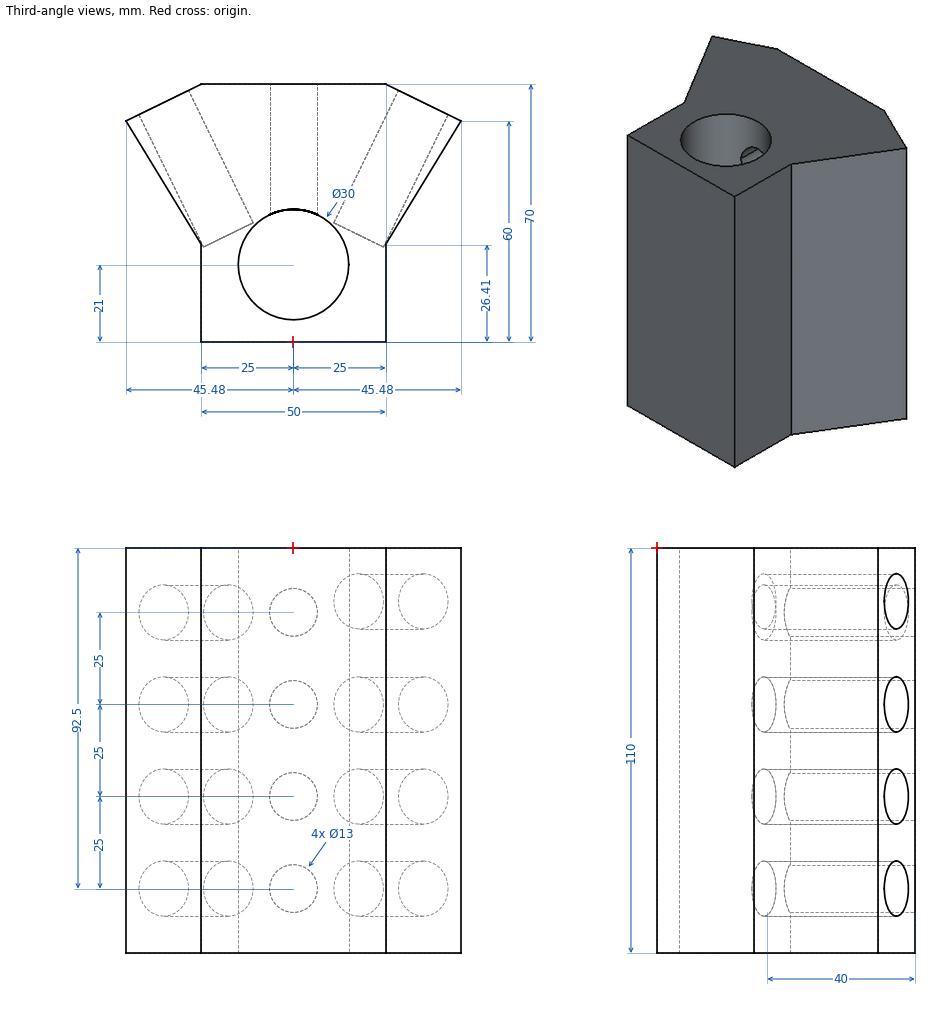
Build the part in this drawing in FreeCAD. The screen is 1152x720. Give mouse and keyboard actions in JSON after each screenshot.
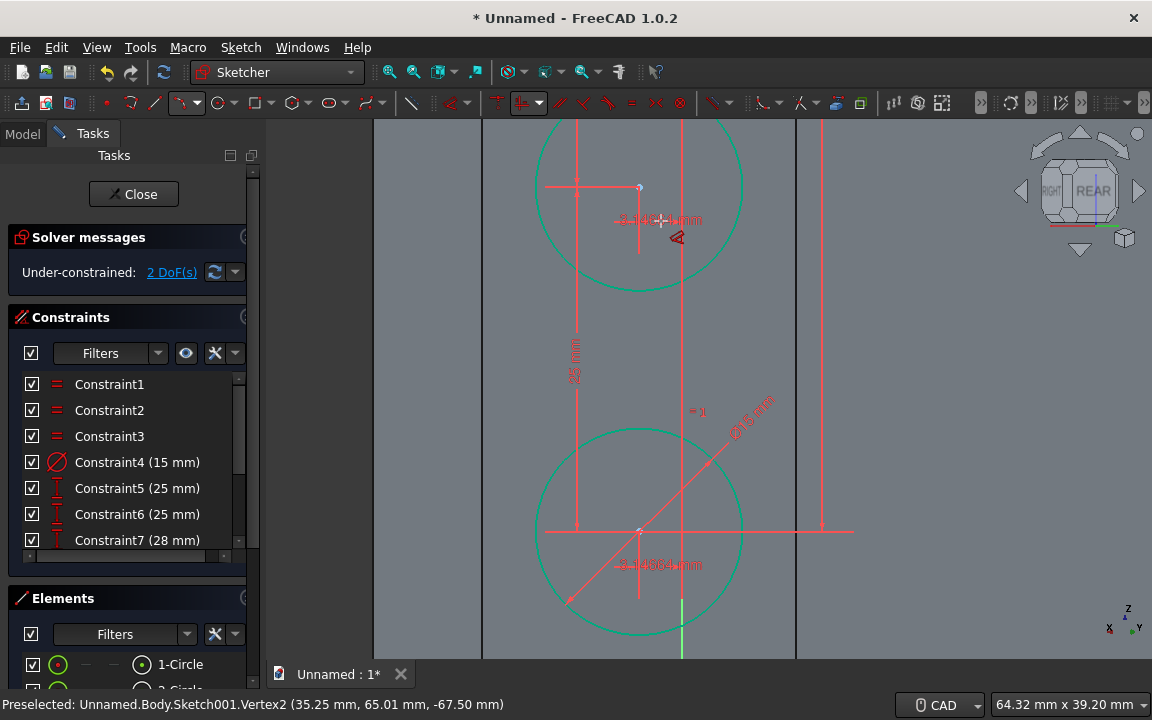
{"action": "scroll", "coordinate": [641, 534], "scroll_direction": "down", "scroll_amount": 7}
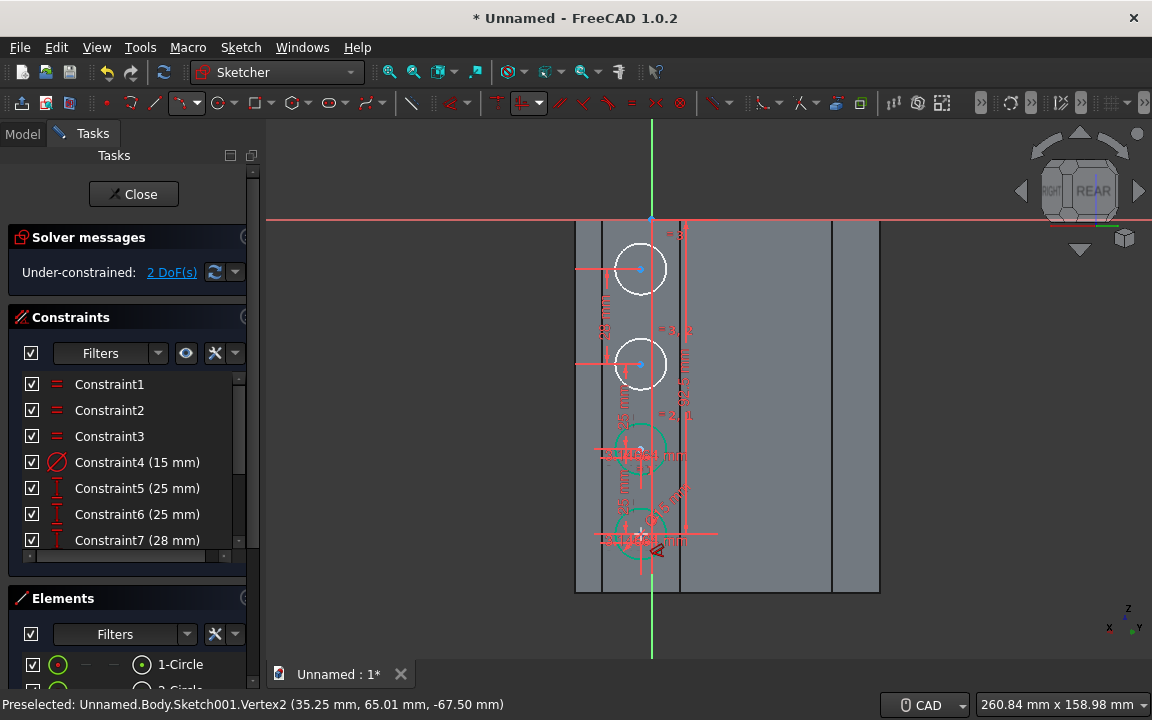
{"action": "scroll", "coordinate": [641, 364], "scroll_direction": "up", "scroll_amount": 7}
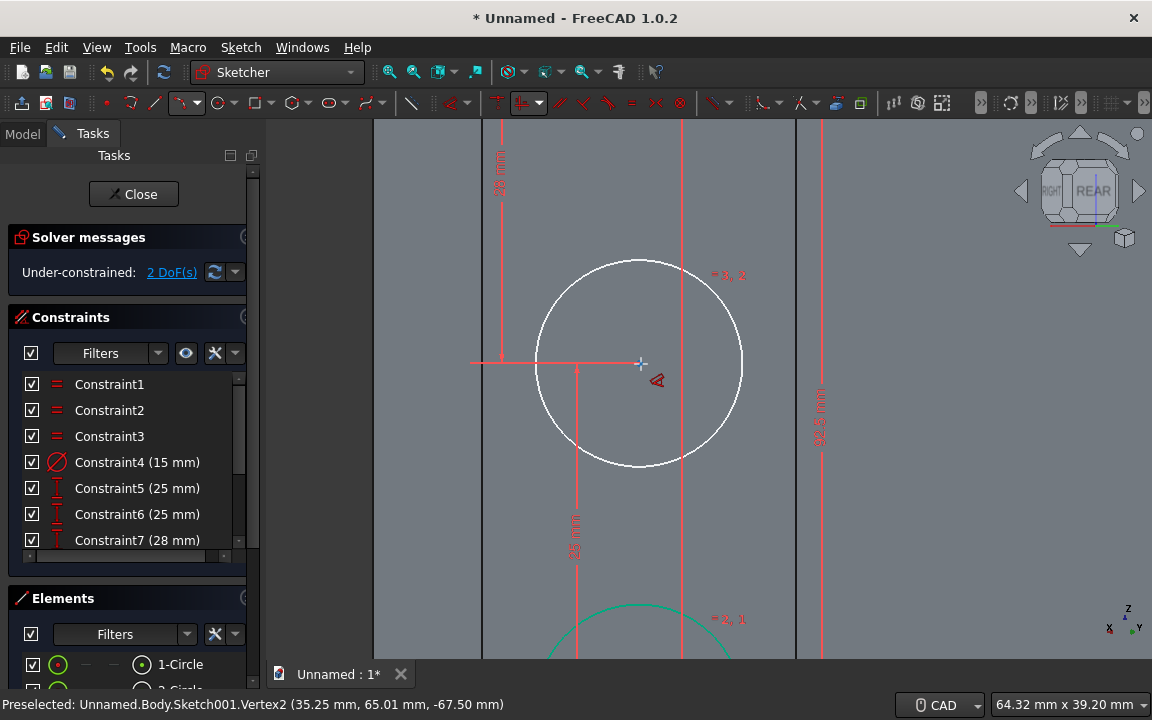
{"action": "left_click", "coordinate": [639, 363]}
{"action": "left_click", "coordinate": [661, 397]}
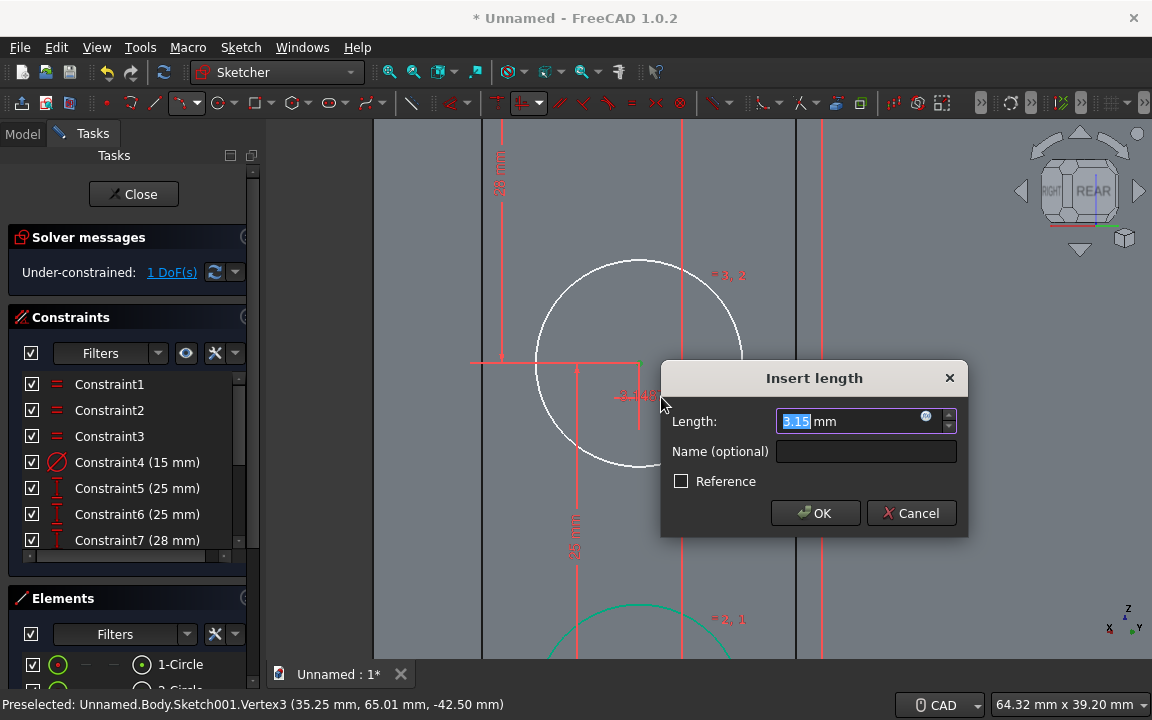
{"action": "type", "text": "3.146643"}
{"action": "key", "text": "Return"}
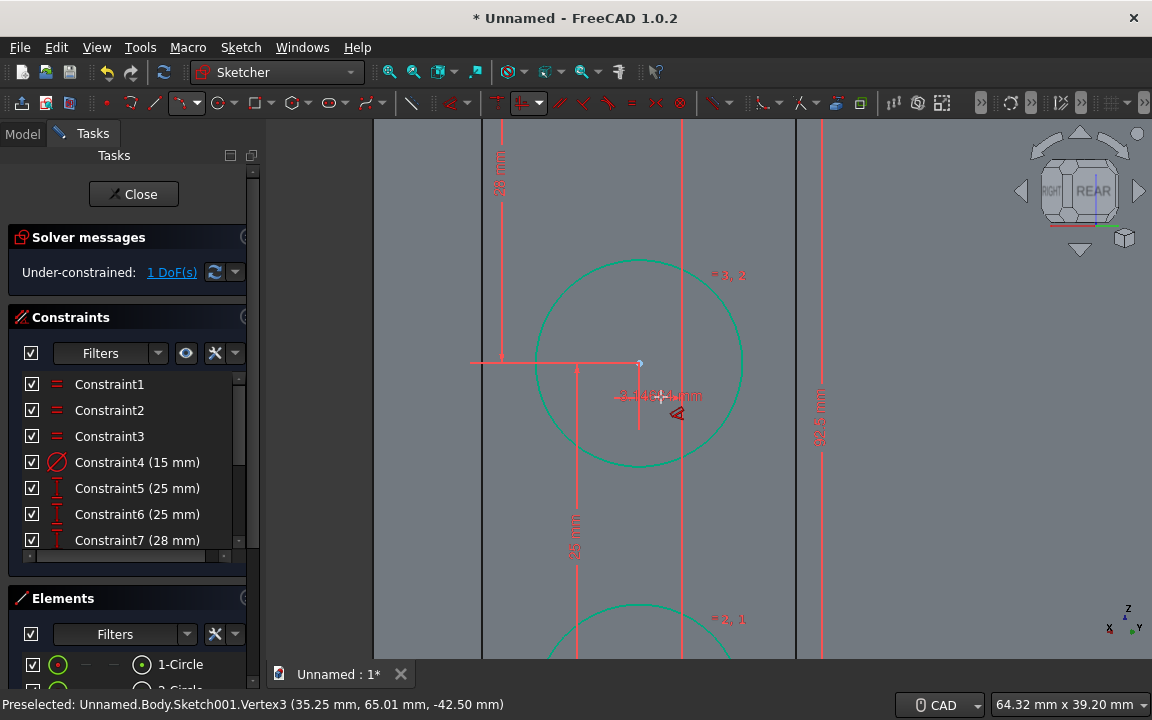
{"action": "scroll", "coordinate": [641, 364], "scroll_direction": "down", "scroll_amount": 7}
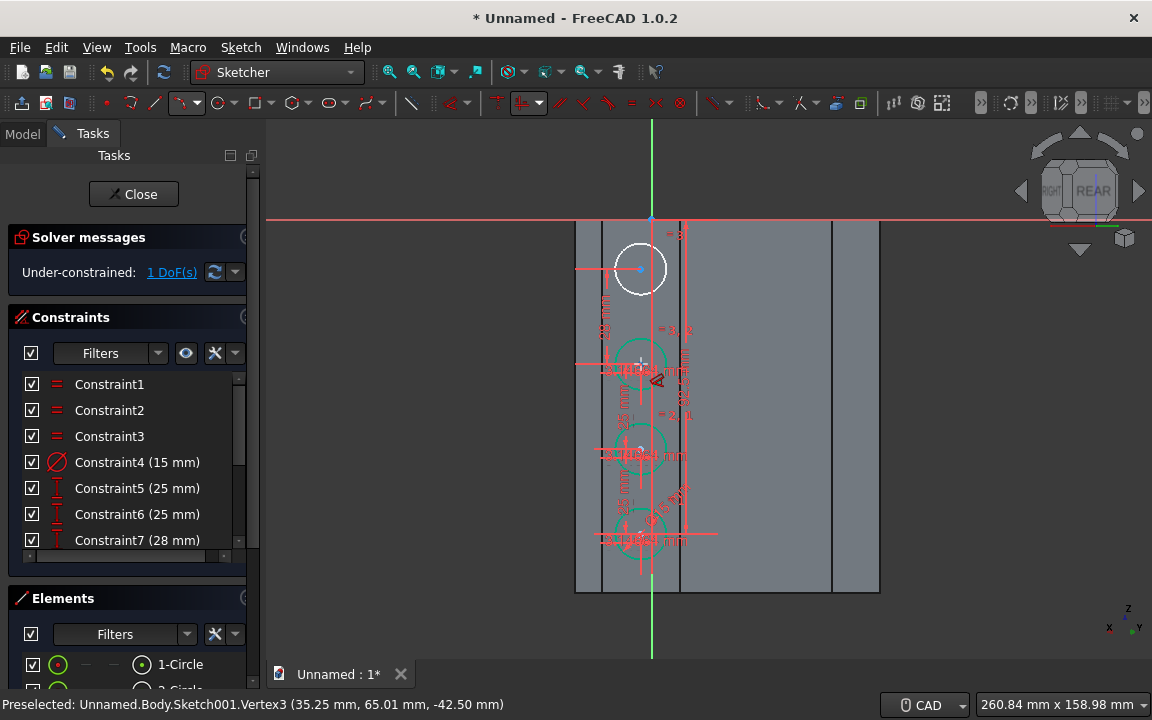
{"action": "scroll", "coordinate": [641, 269], "scroll_direction": "up", "scroll_amount": 7}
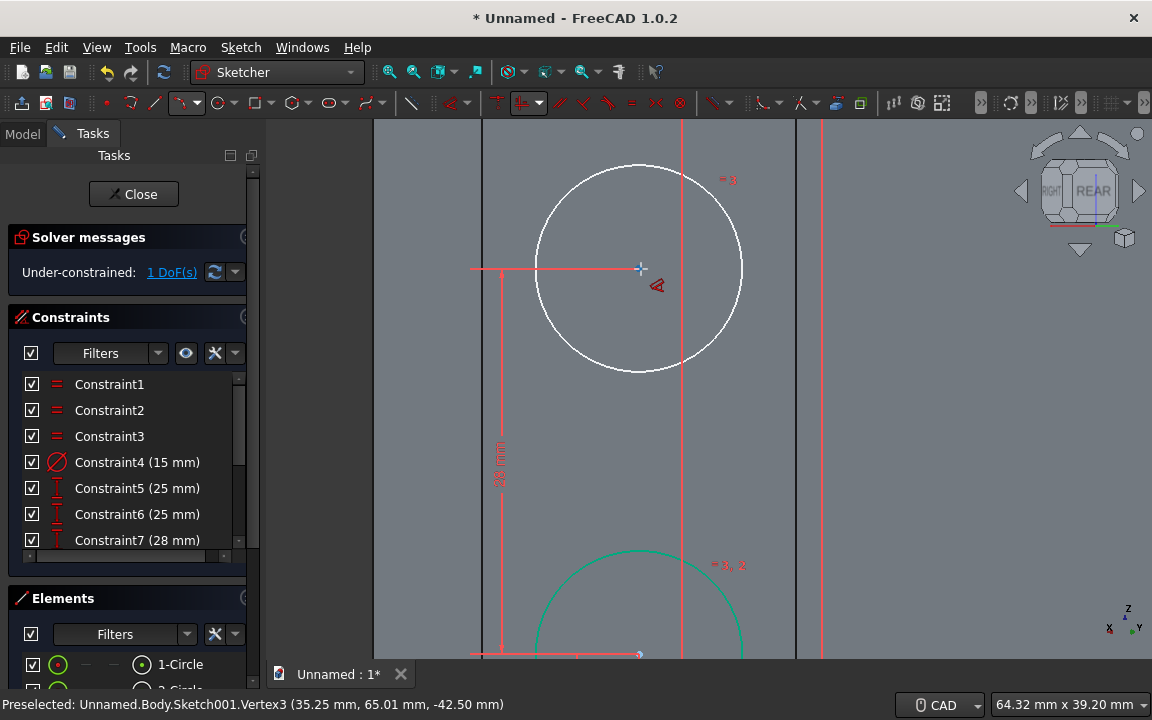
{"action": "left_click", "coordinate": [639, 269]}
{"action": "left_click", "coordinate": [661, 303]}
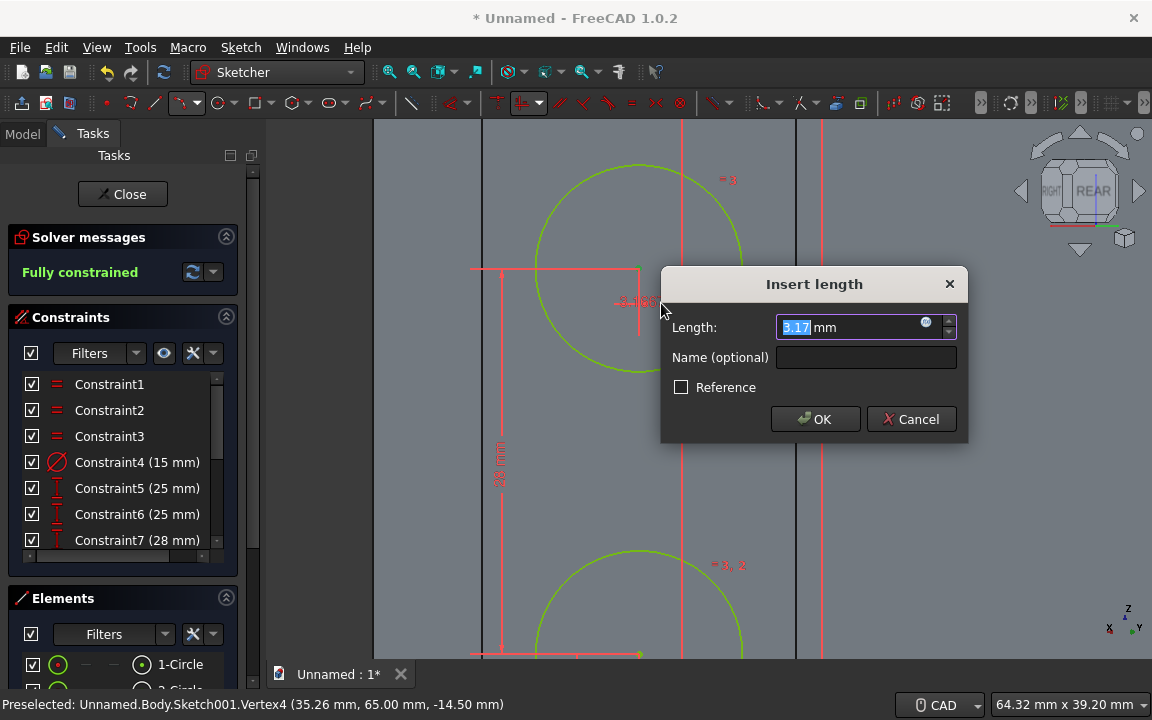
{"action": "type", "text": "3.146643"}
{"action": "key", "text": "Return"}
{"action": "key", "text": "Escape"}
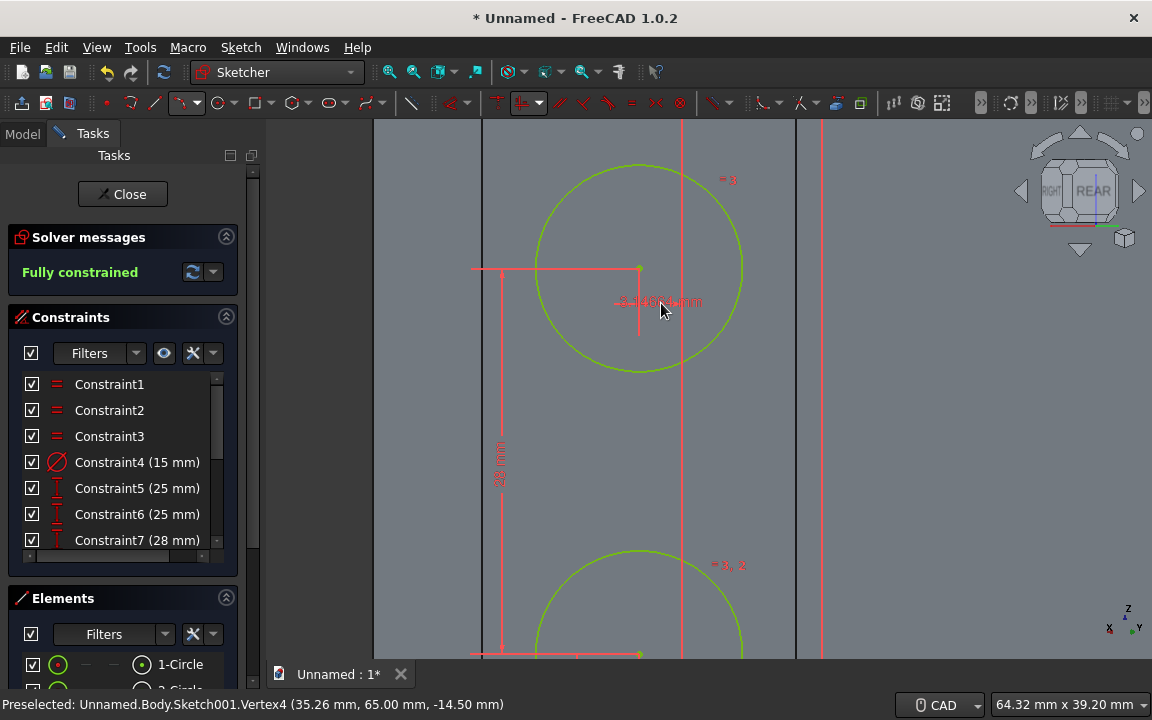
{"action": "left_click", "coordinate": [123, 194]}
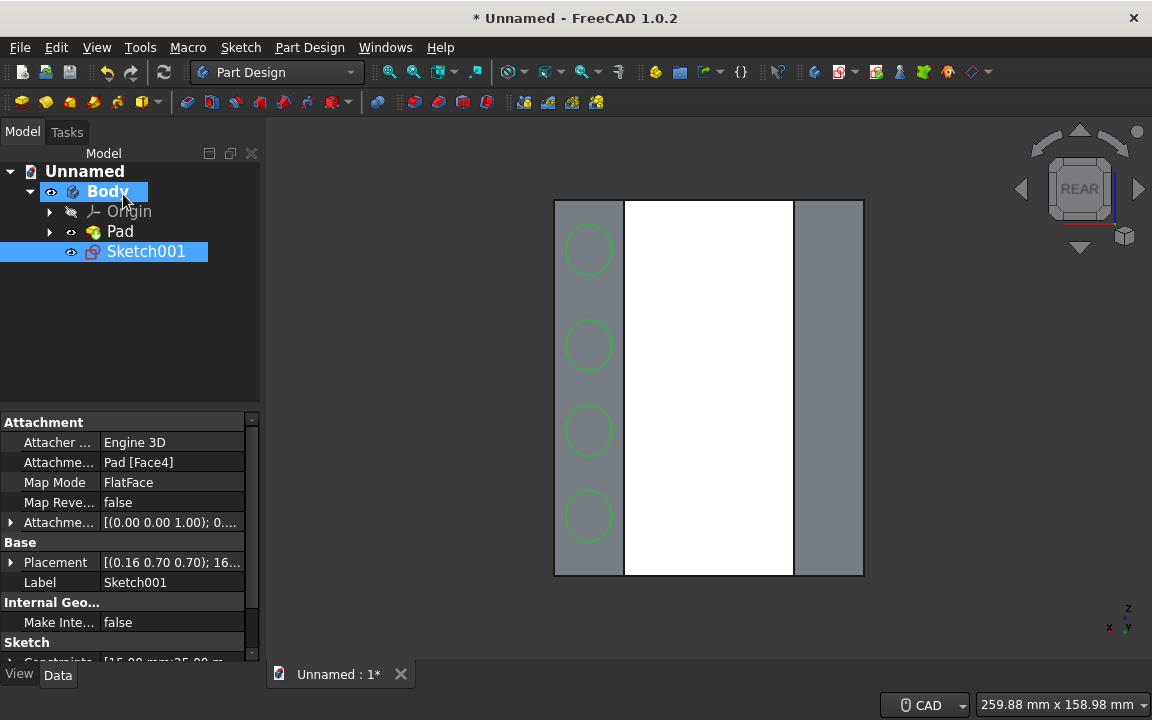
{"action": "left_click", "coordinate": [188, 102]}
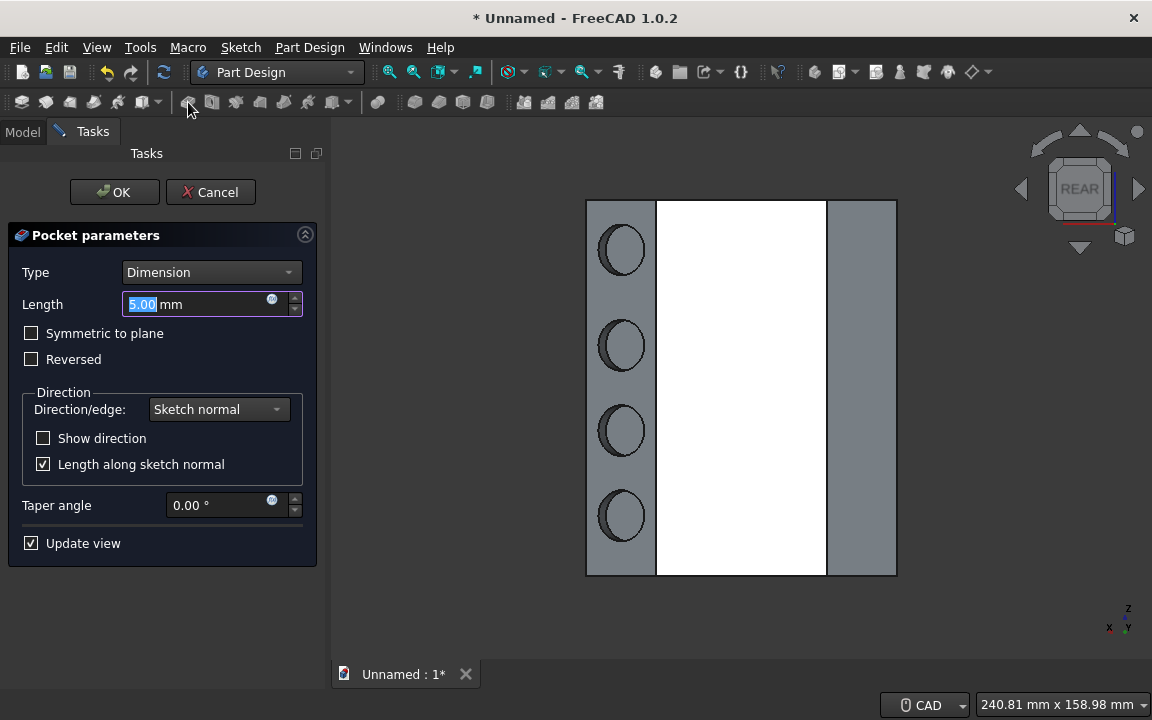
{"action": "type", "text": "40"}
{"action": "key", "text": "Tab"}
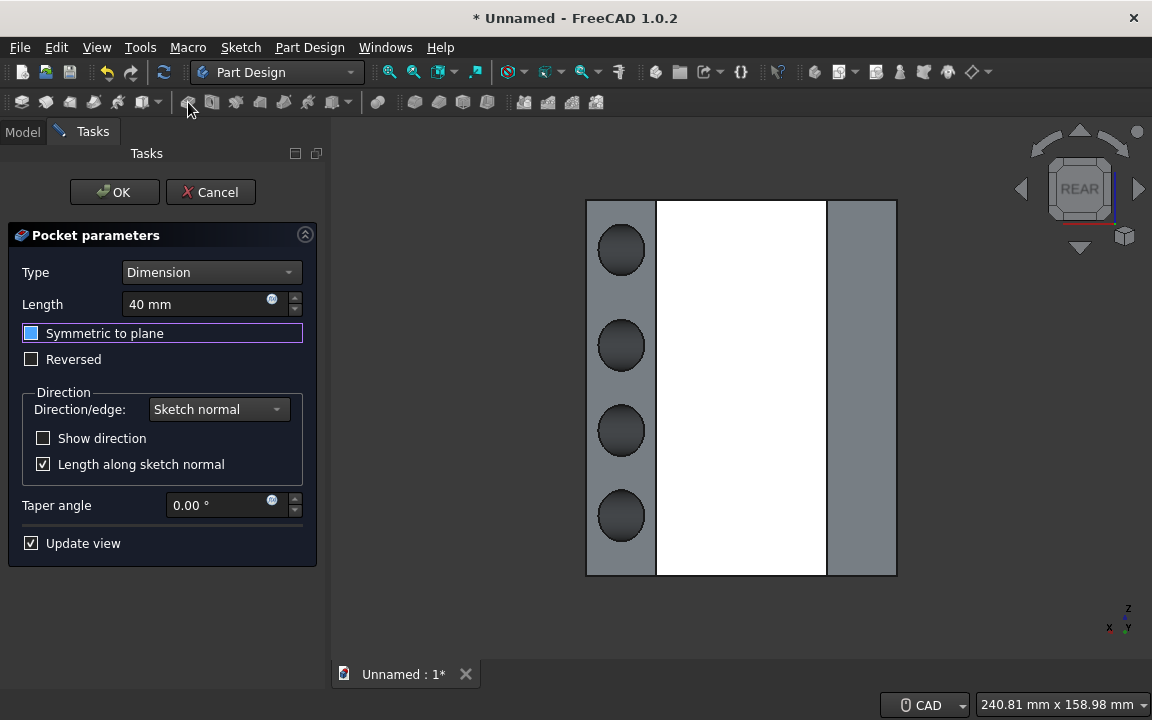
{"action": "left_click", "coordinate": [115, 192]}